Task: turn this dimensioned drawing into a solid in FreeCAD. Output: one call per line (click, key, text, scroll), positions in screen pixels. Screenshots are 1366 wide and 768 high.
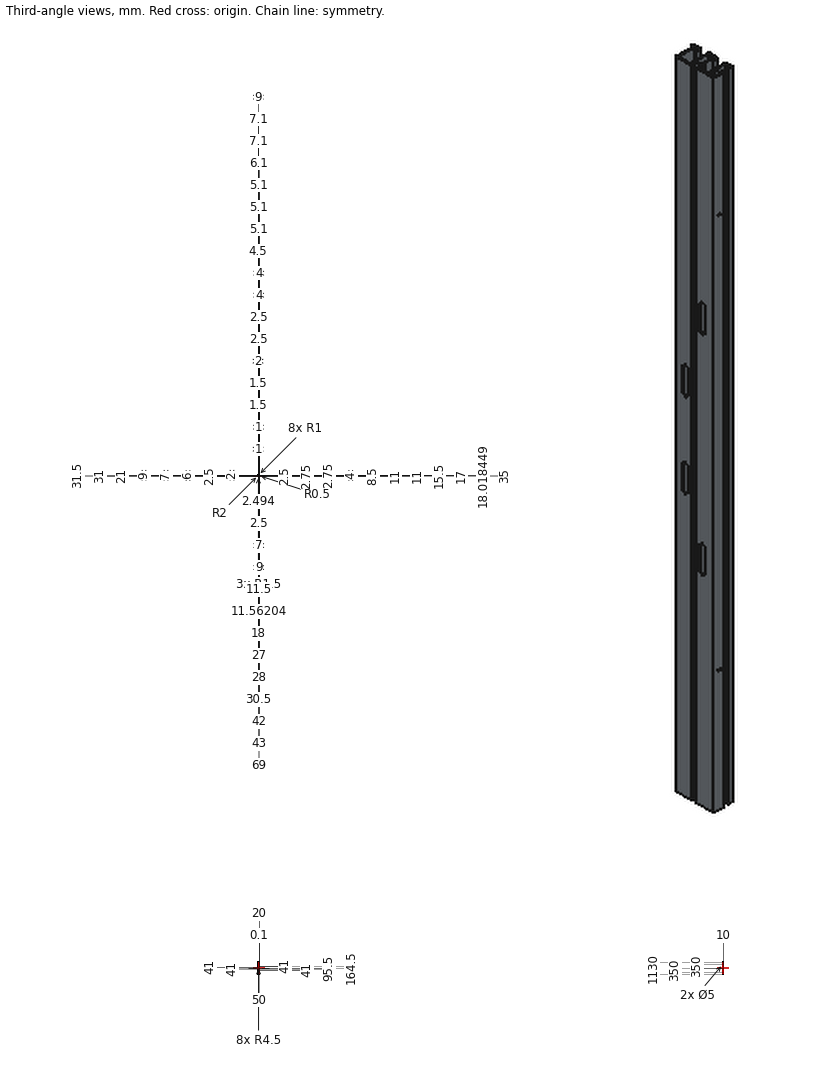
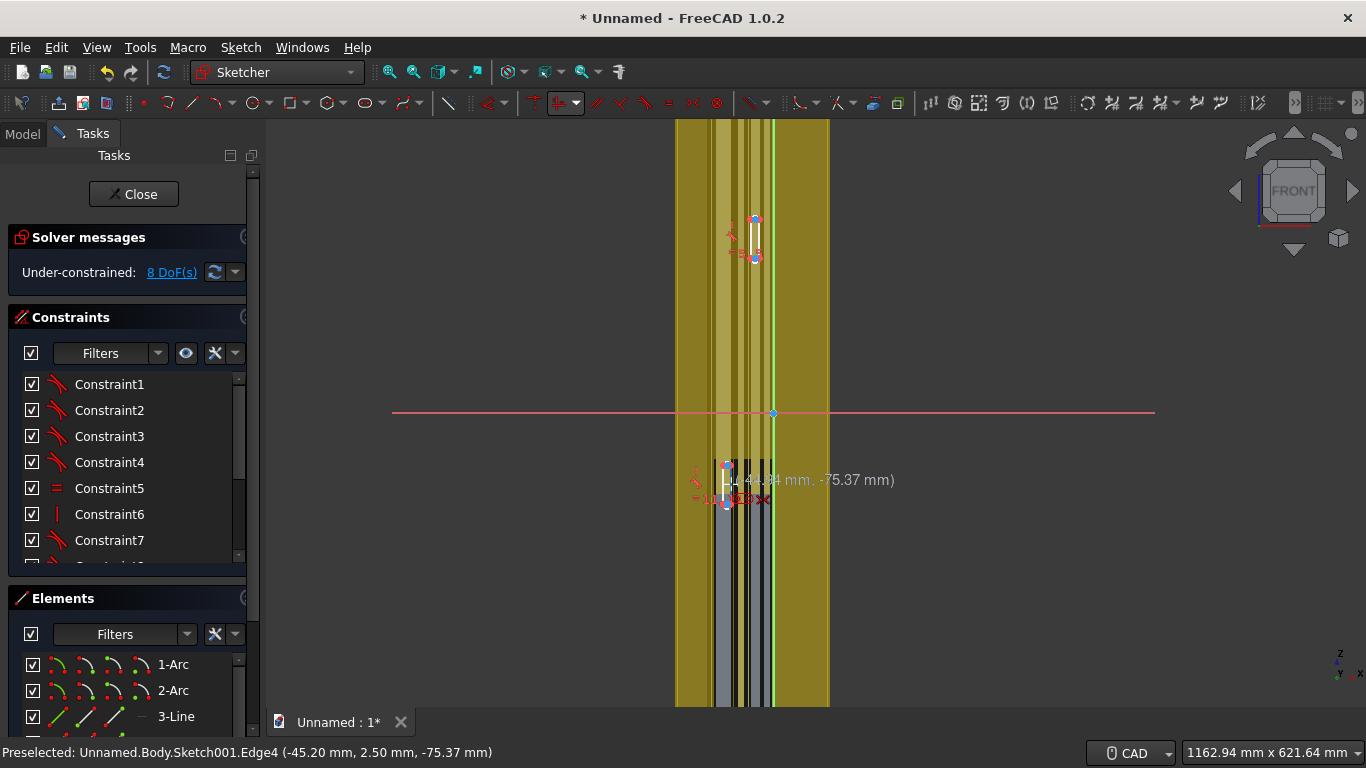
scroll(727, 362, up, 9)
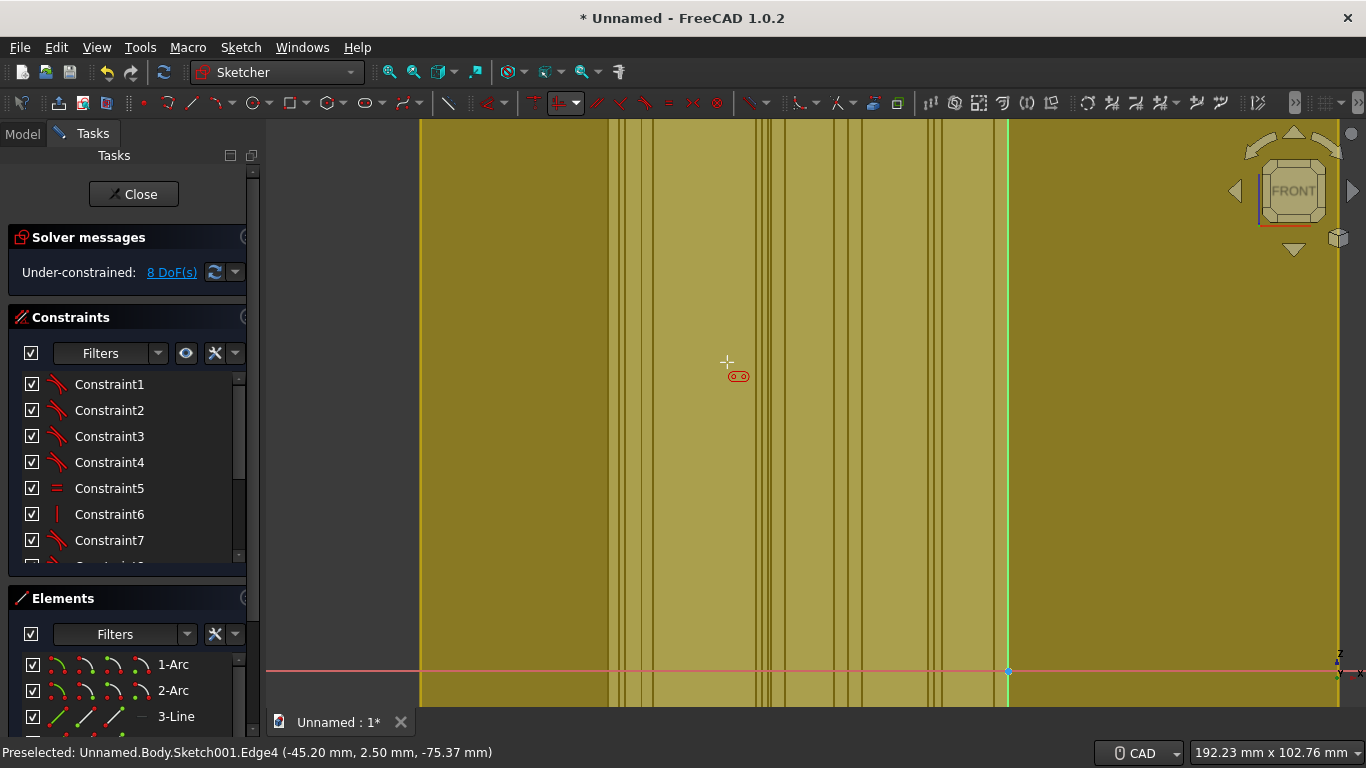
scroll(727, 362, down, 9)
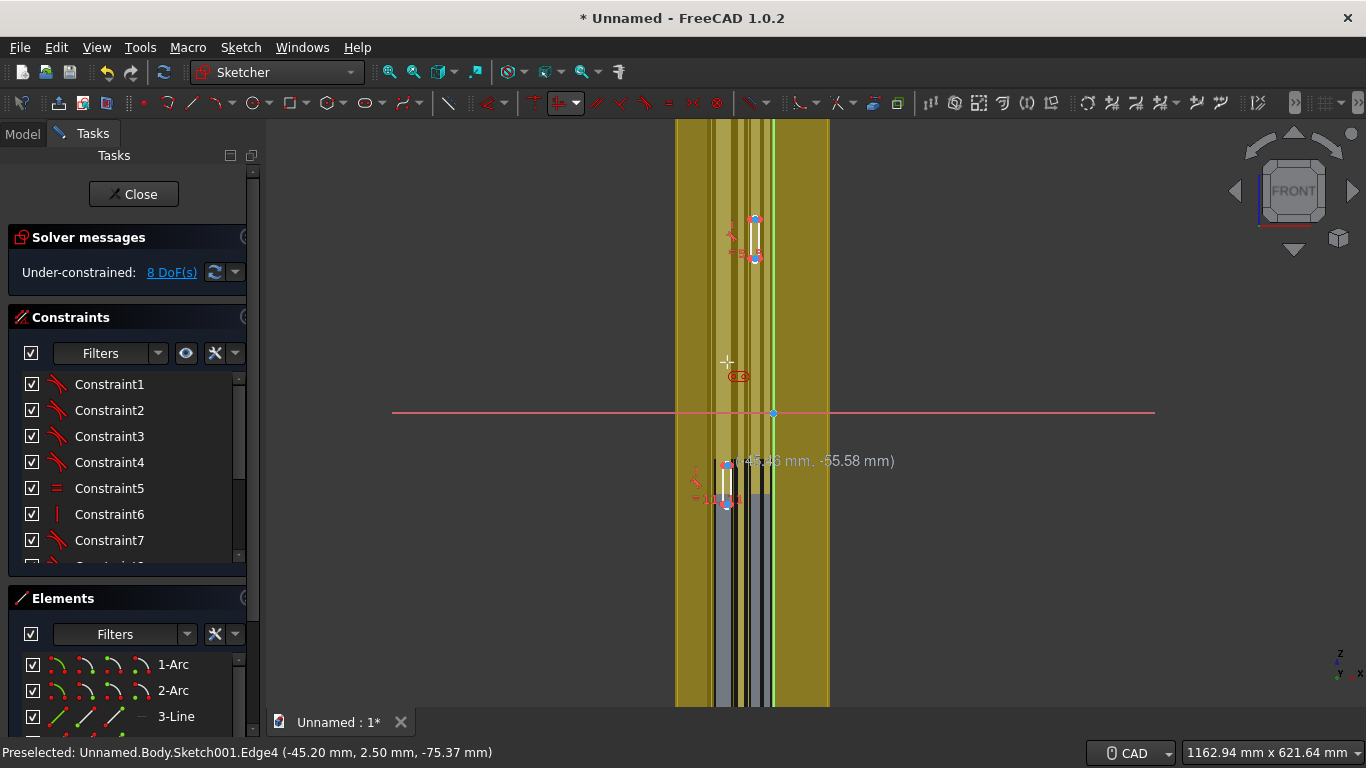
click(727, 362)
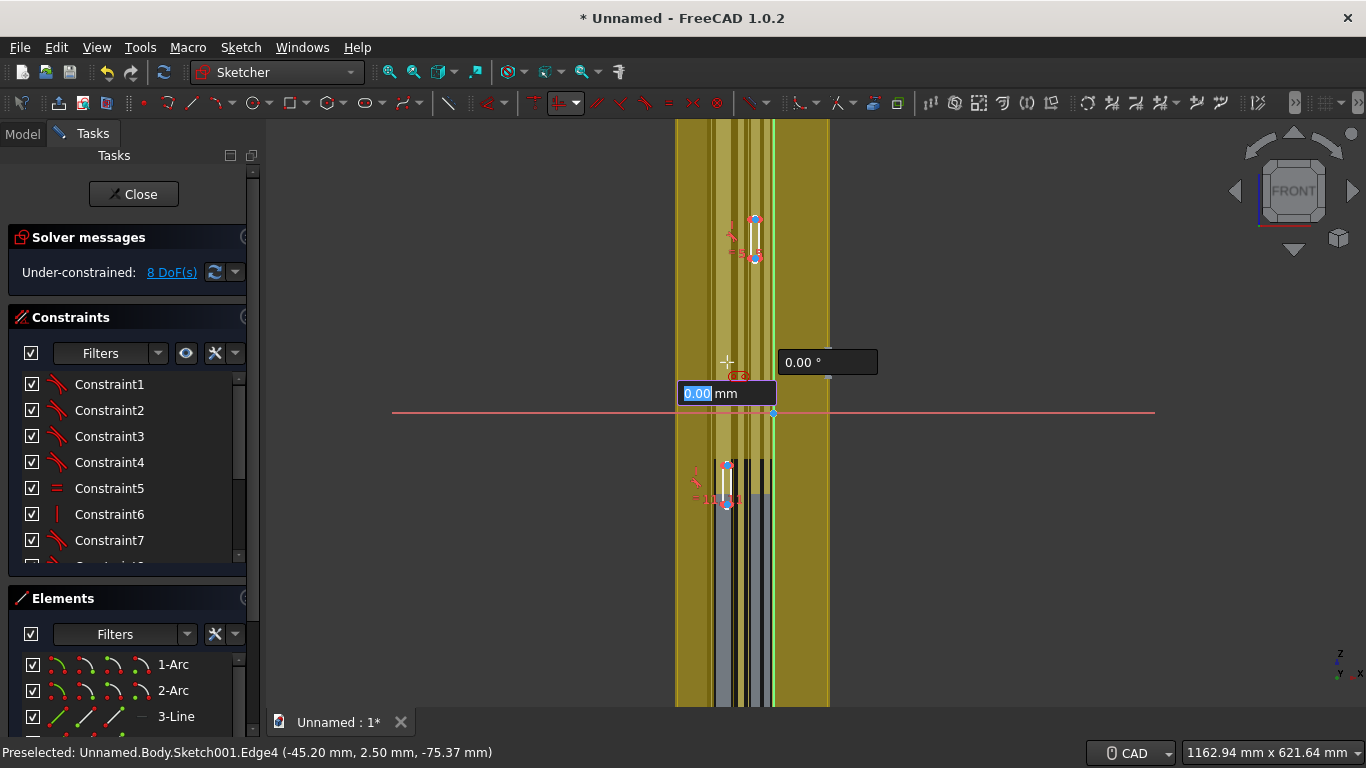
click(727, 323)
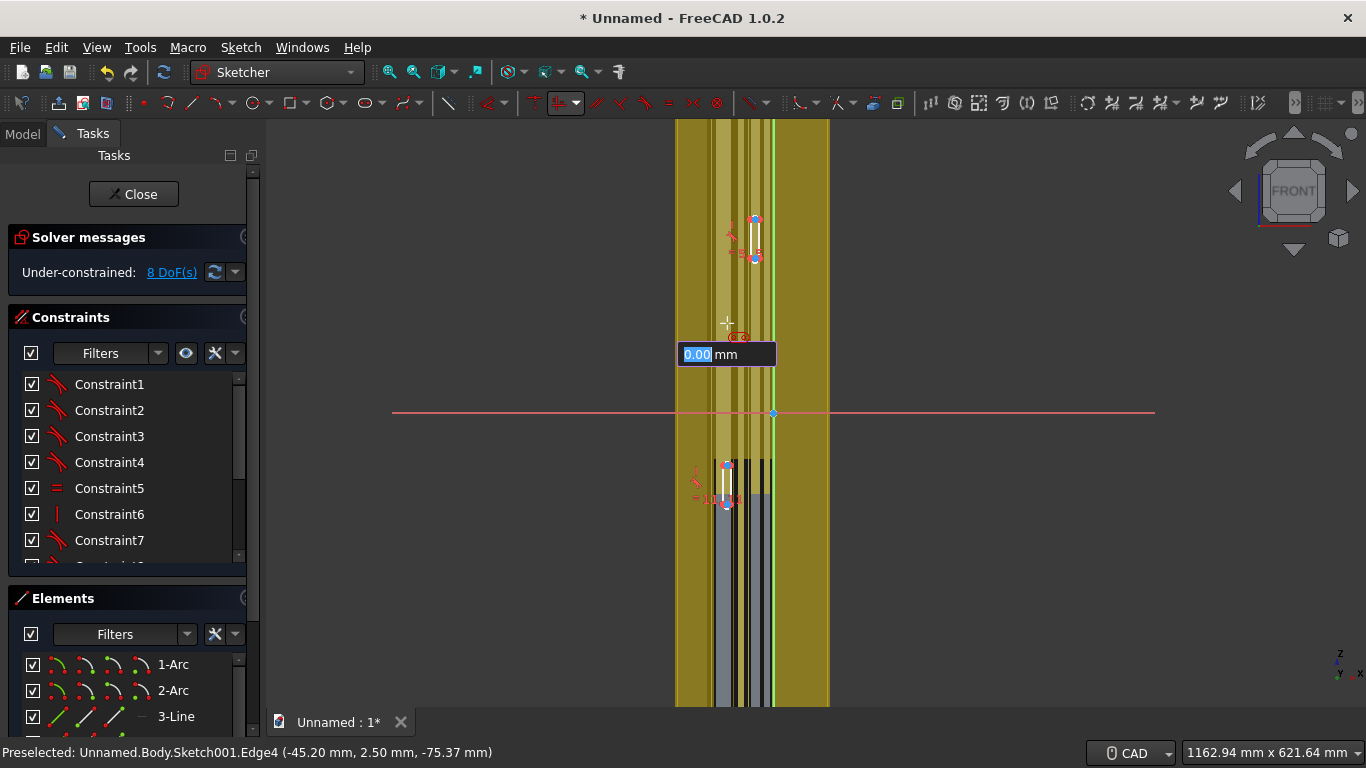
scroll(731, 342, up, 7)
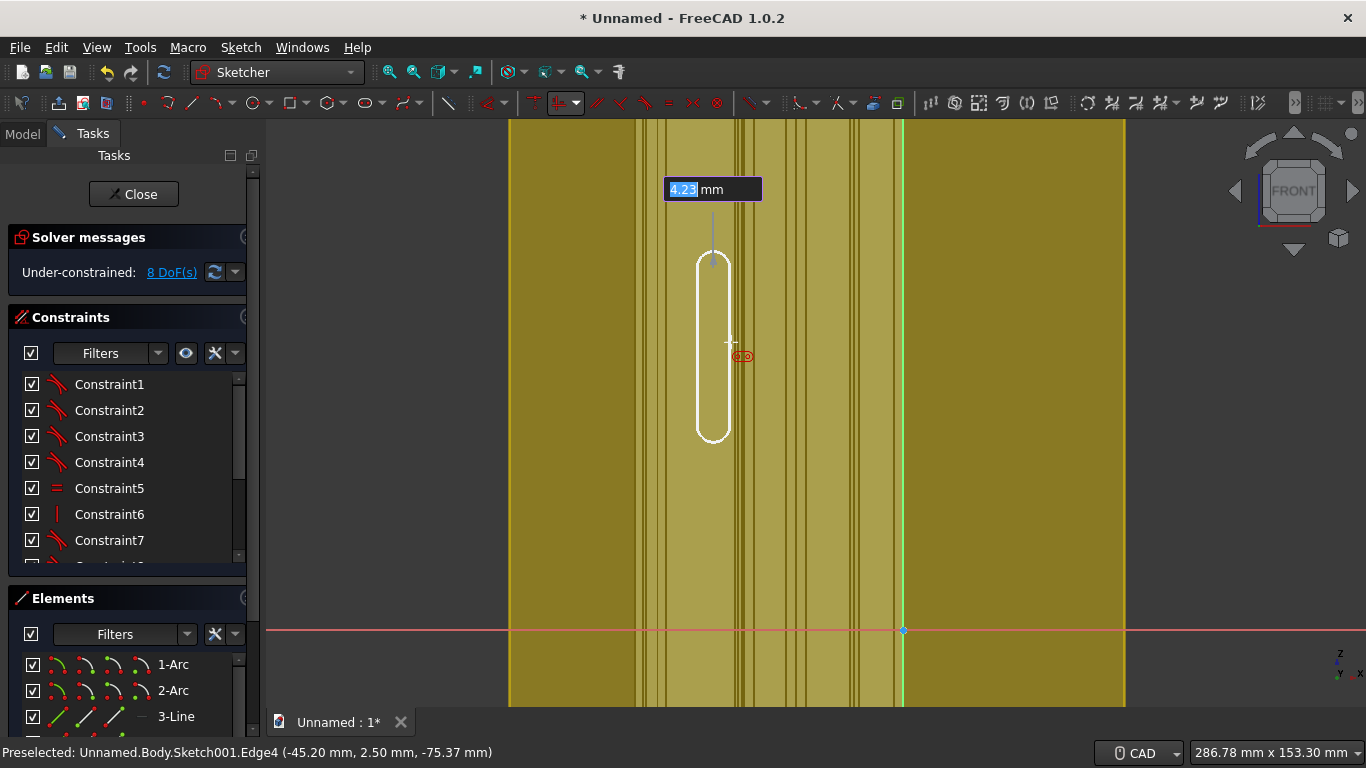
click(729, 343)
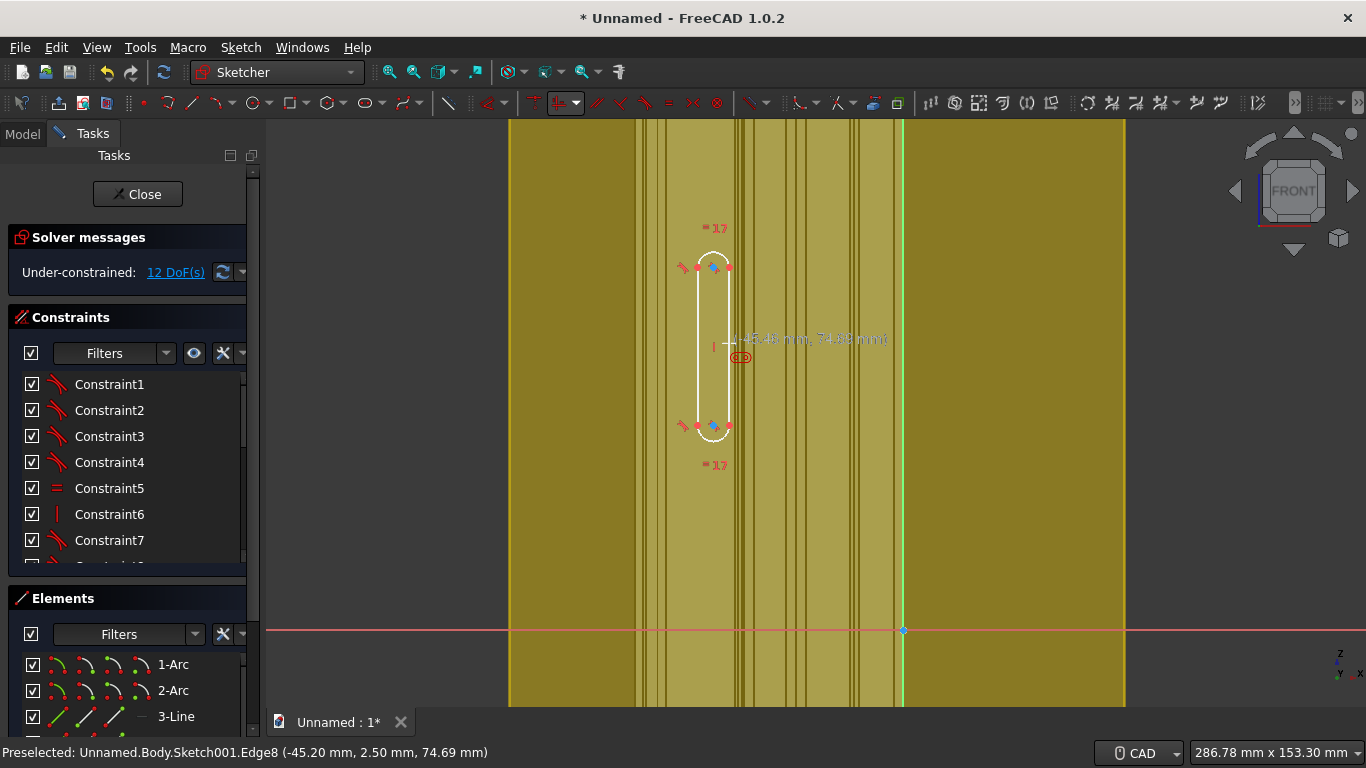
scroll(731, 342, down, 7)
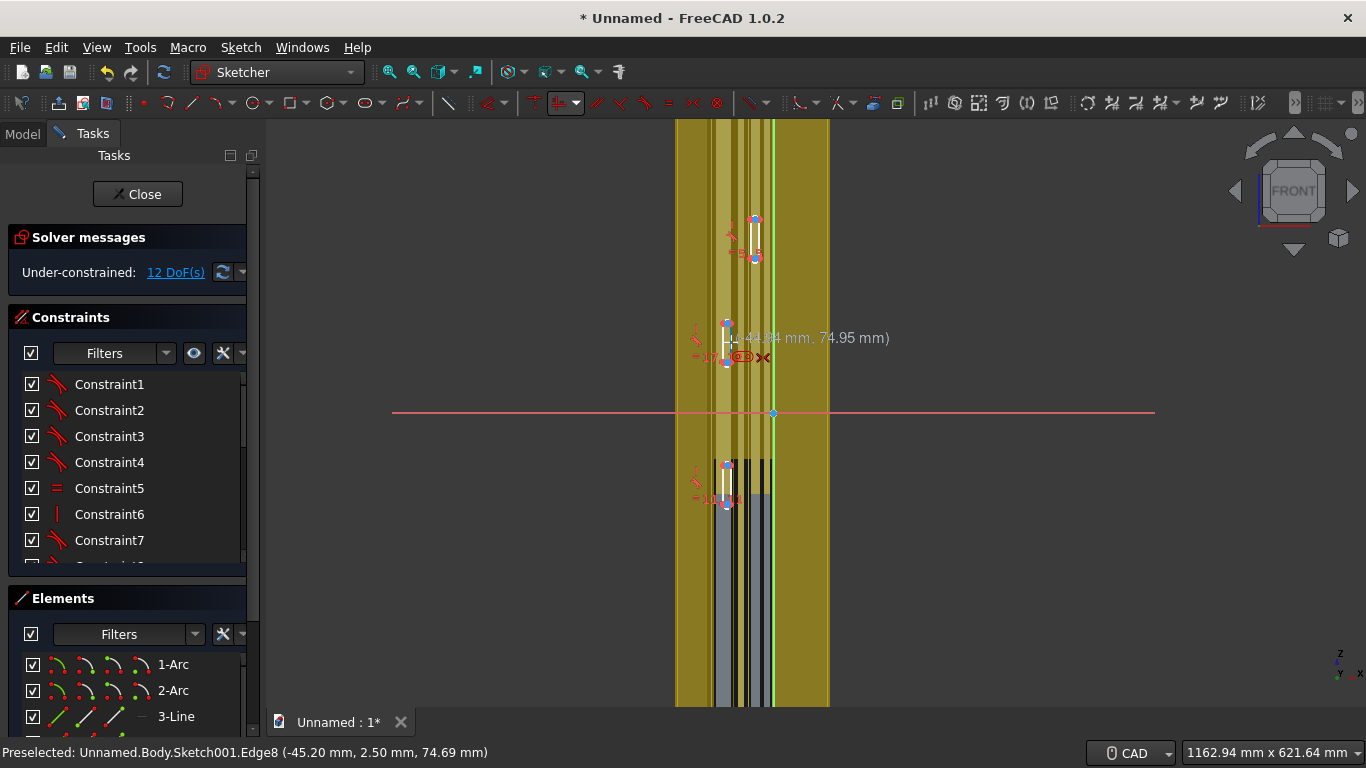
scroll(755, 608, up, 9)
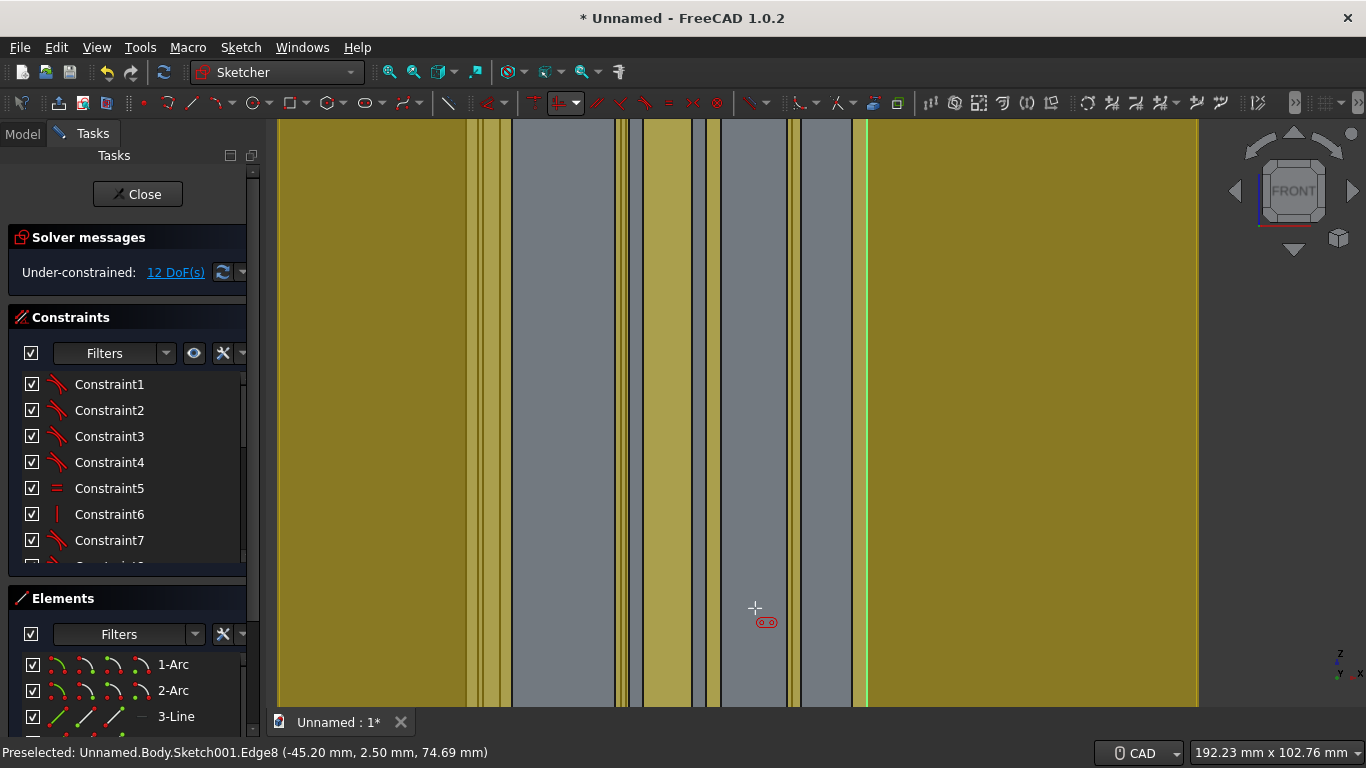
scroll(755, 608, down, 9)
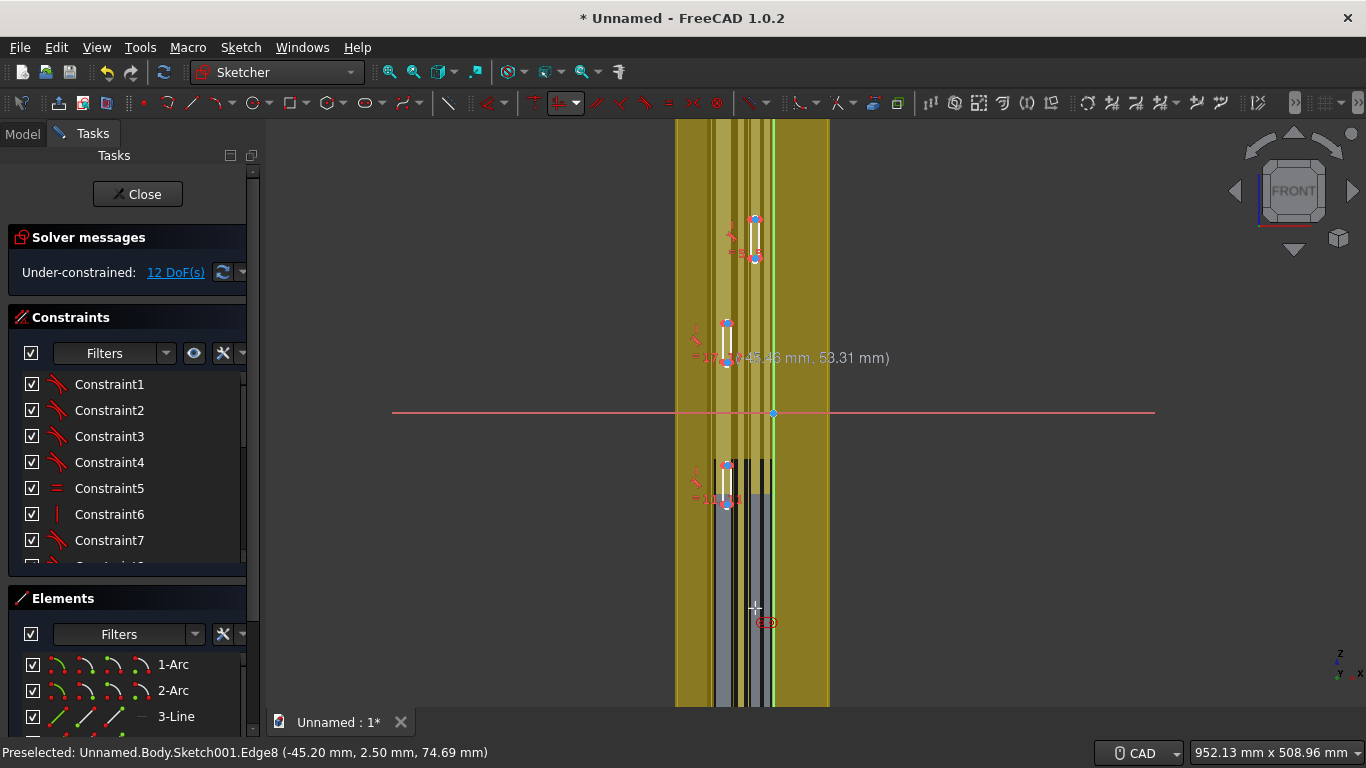
click(755, 608)